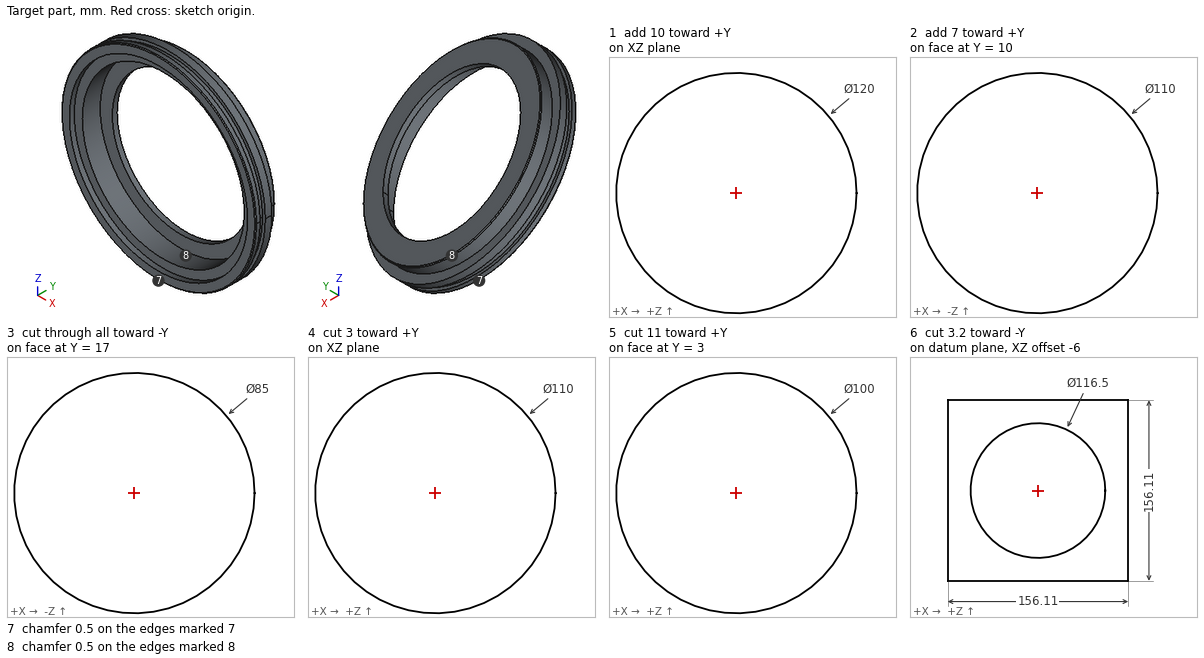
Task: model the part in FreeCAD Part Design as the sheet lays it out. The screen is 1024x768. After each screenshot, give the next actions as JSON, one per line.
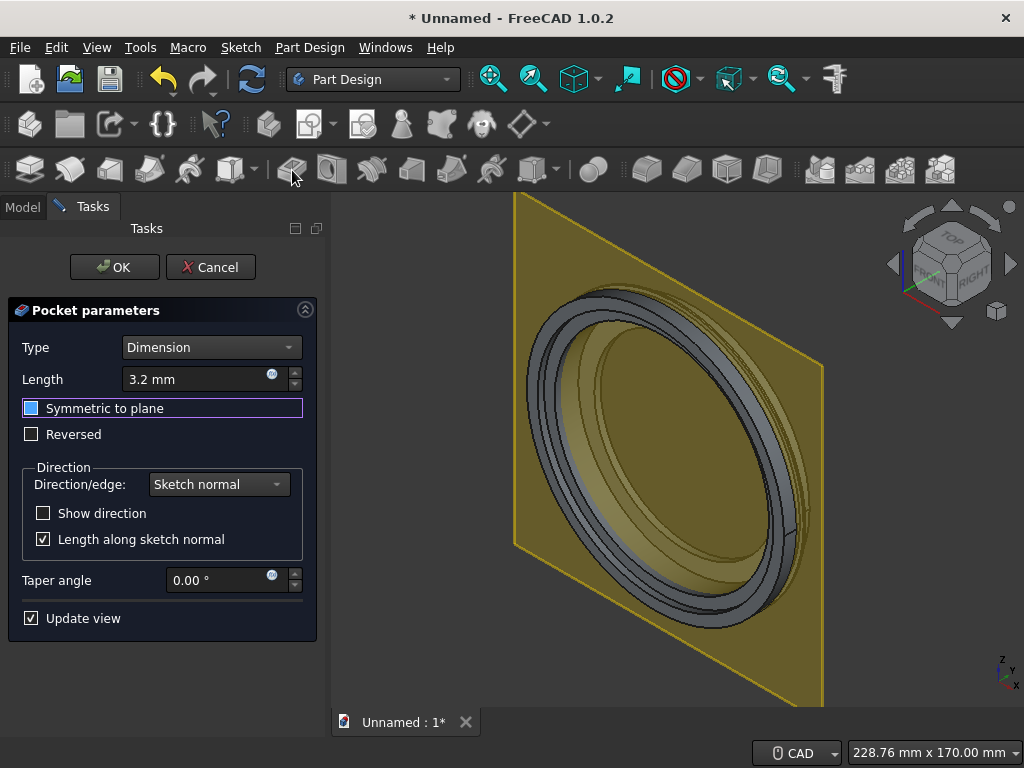
{"action": "left_click", "coordinate": [30, 434]}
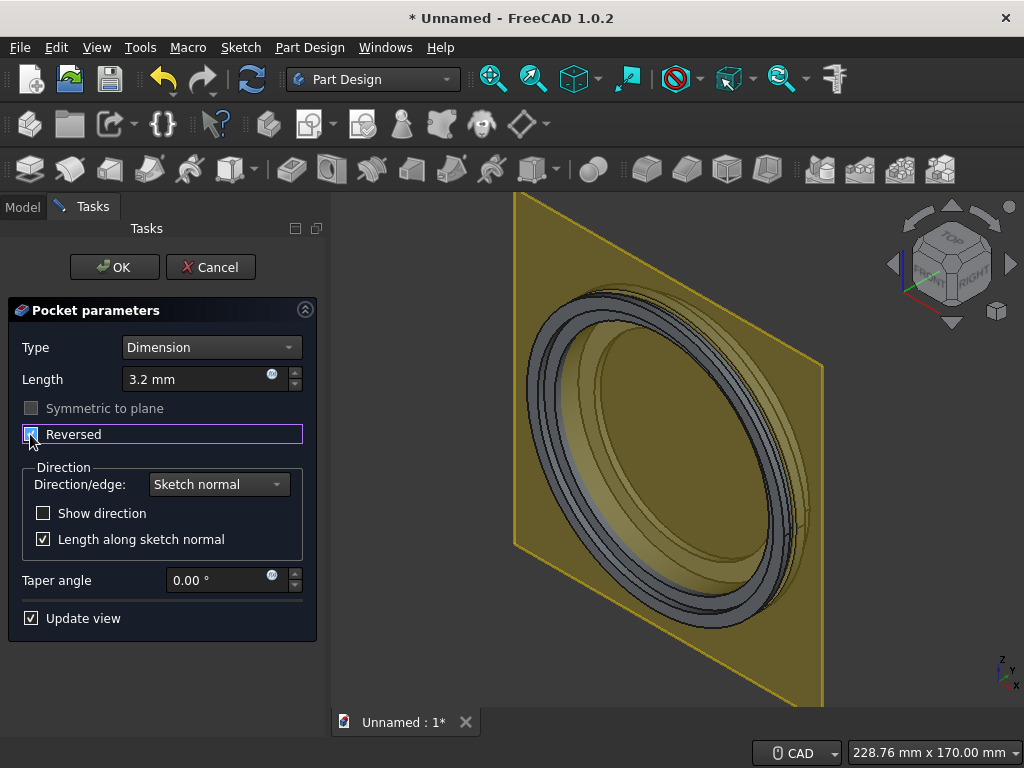
{"action": "left_click", "coordinate": [115, 267]}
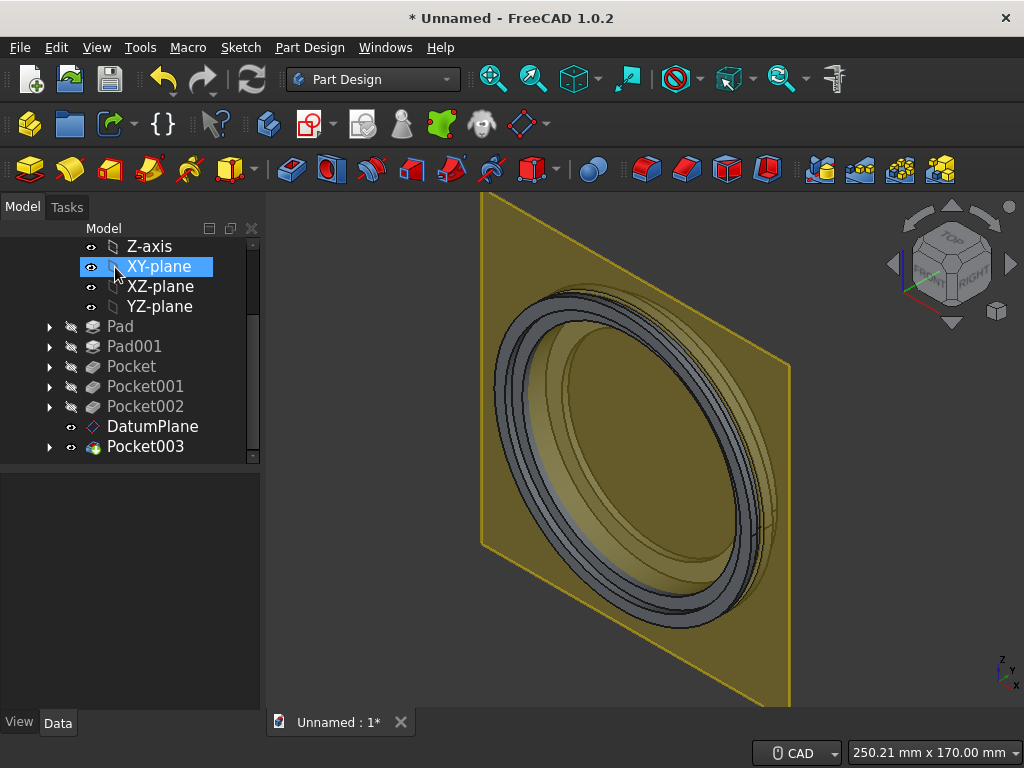
{"action": "left_click", "coordinate": [116, 427]}
{"action": "key", "text": "space"}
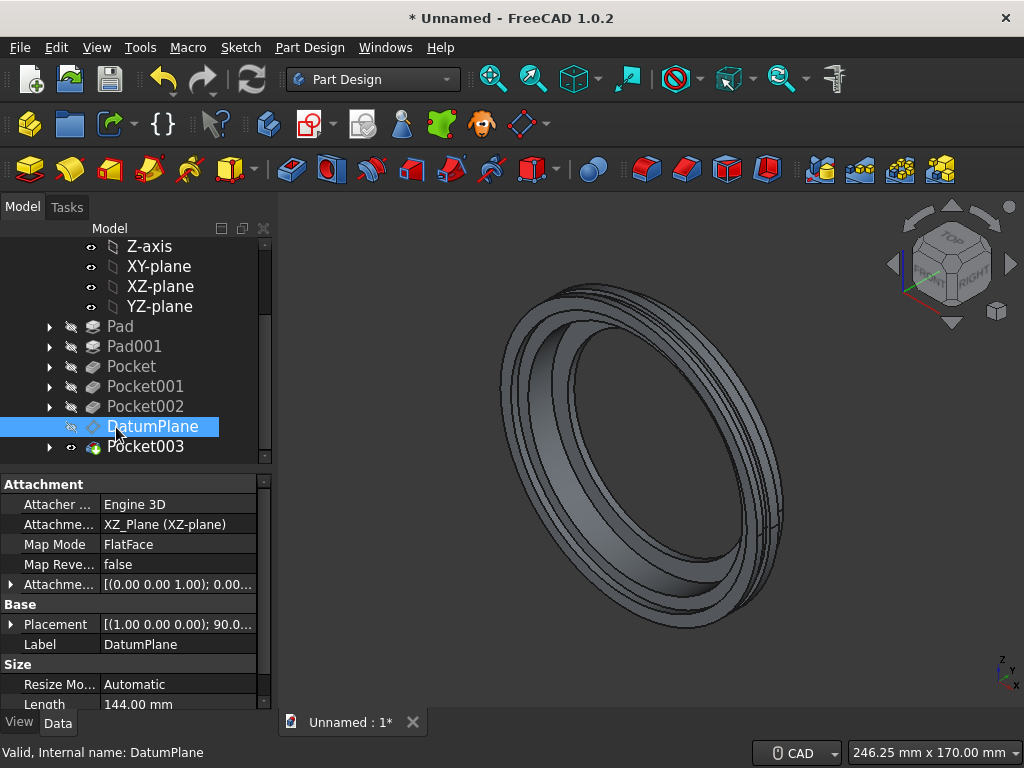
{"action": "left_click", "coordinate": [589, 297]}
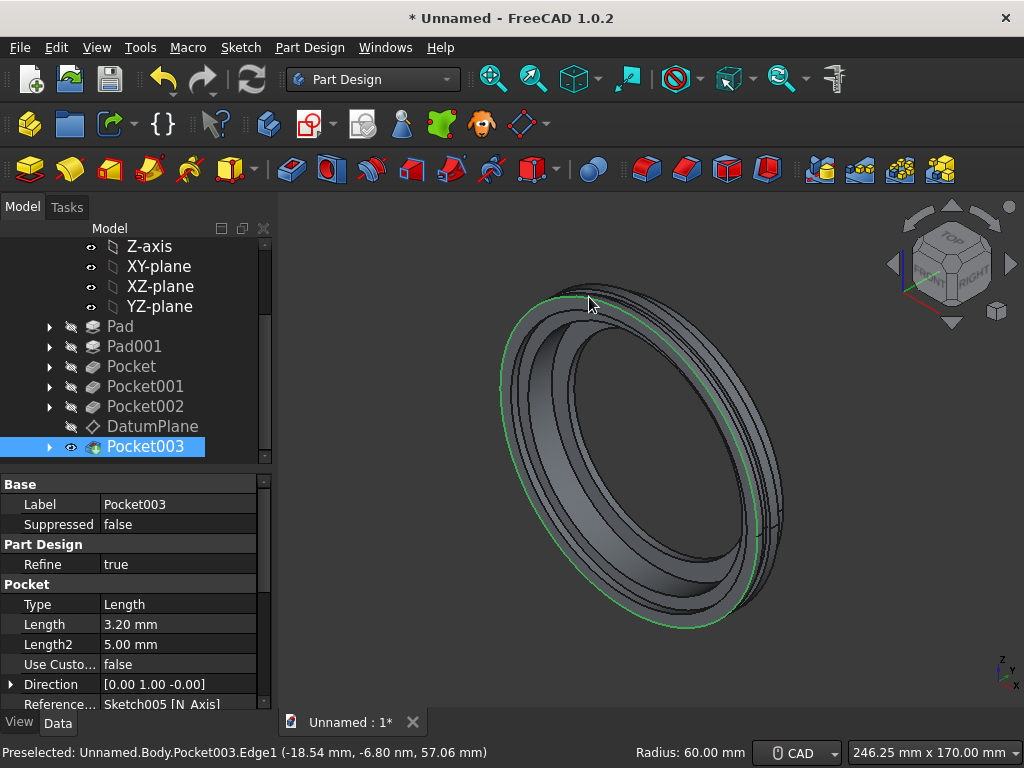
{"action": "left_click", "coordinate": [688, 170]}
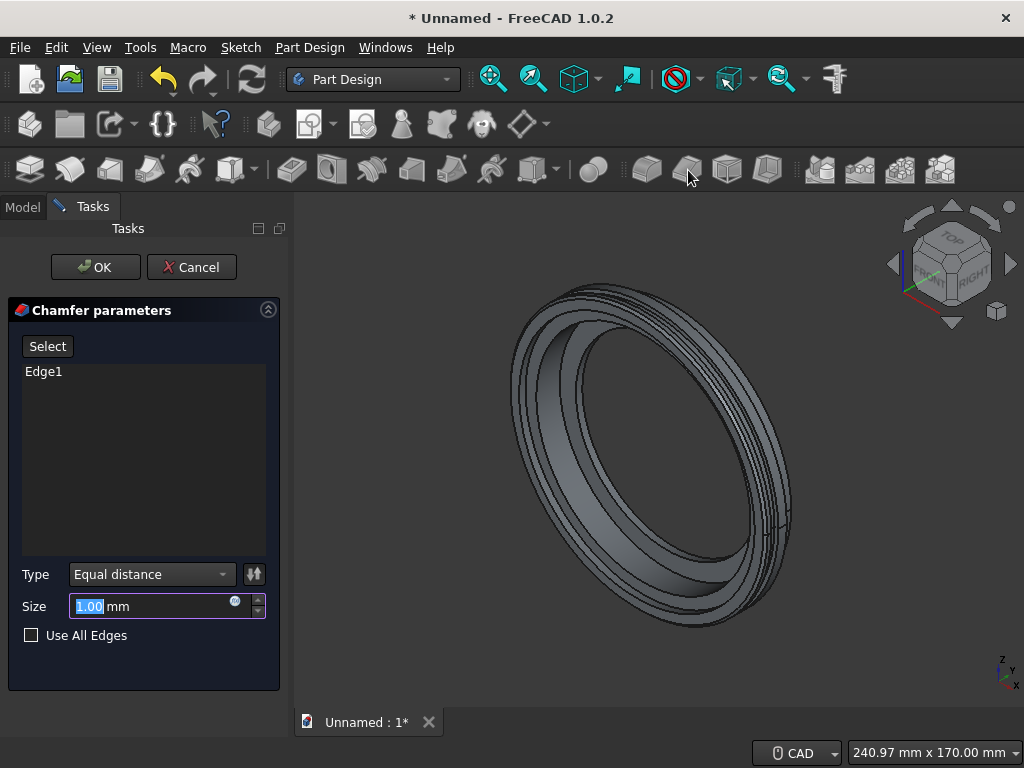
{"action": "type", "text": "0.5"}
{"action": "key", "text": "Tab"}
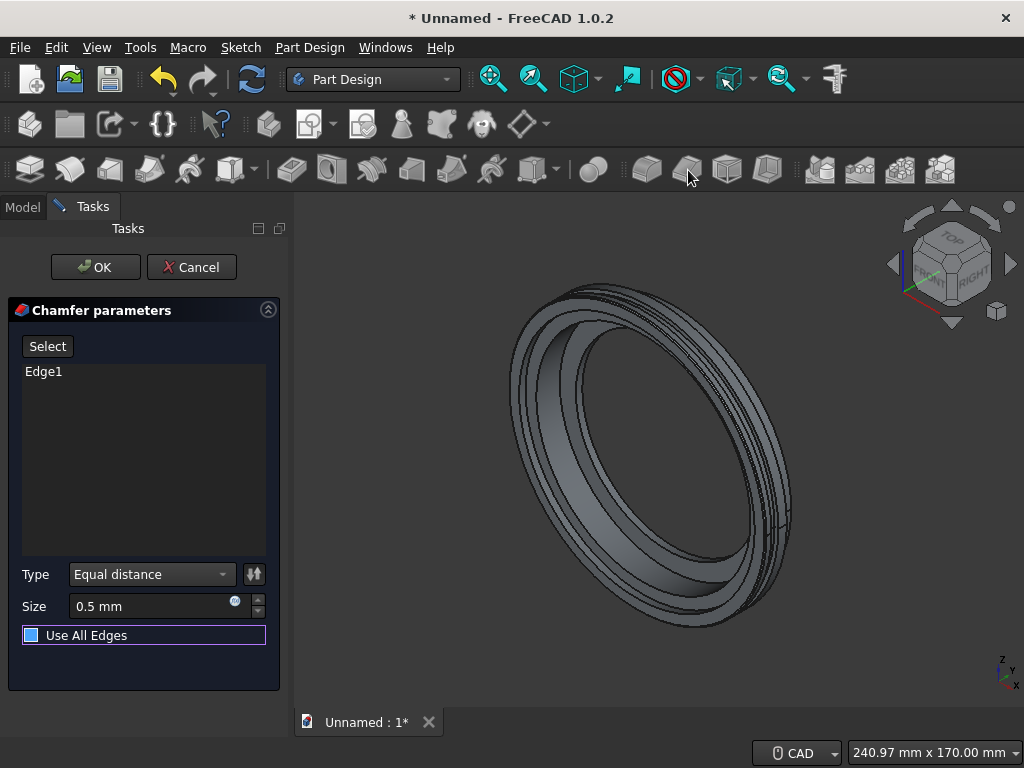
{"action": "left_click", "coordinate": [96, 267]}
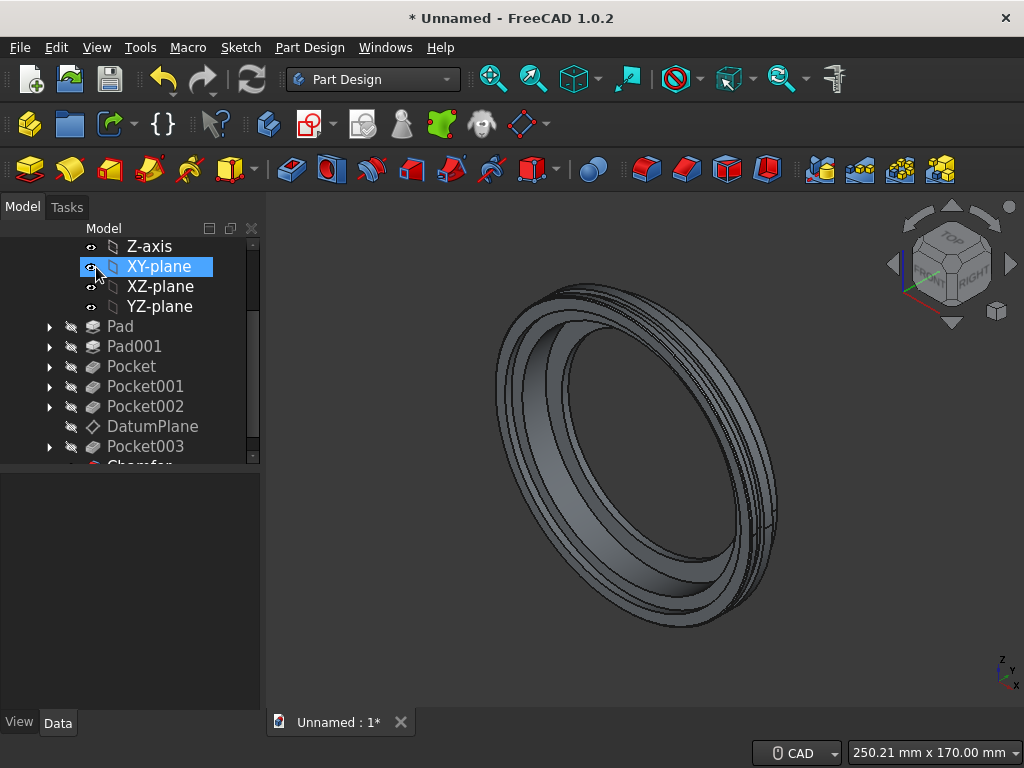
{"action": "key", "text": "2"}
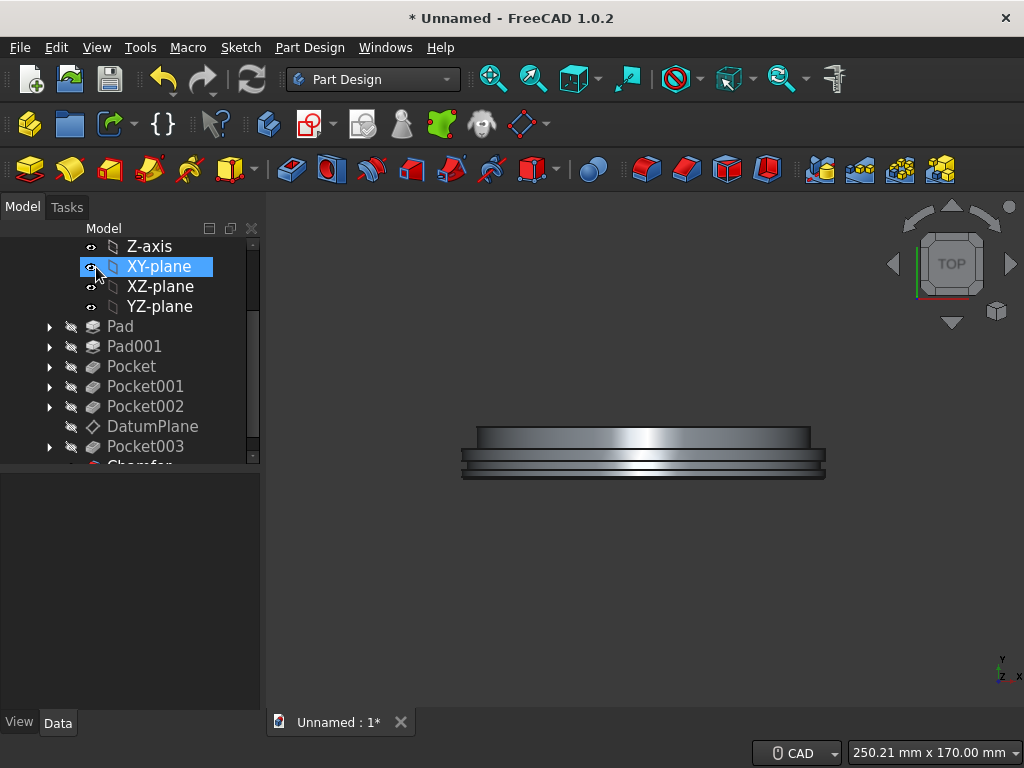
{"action": "left_click", "coordinate": [508, 426]}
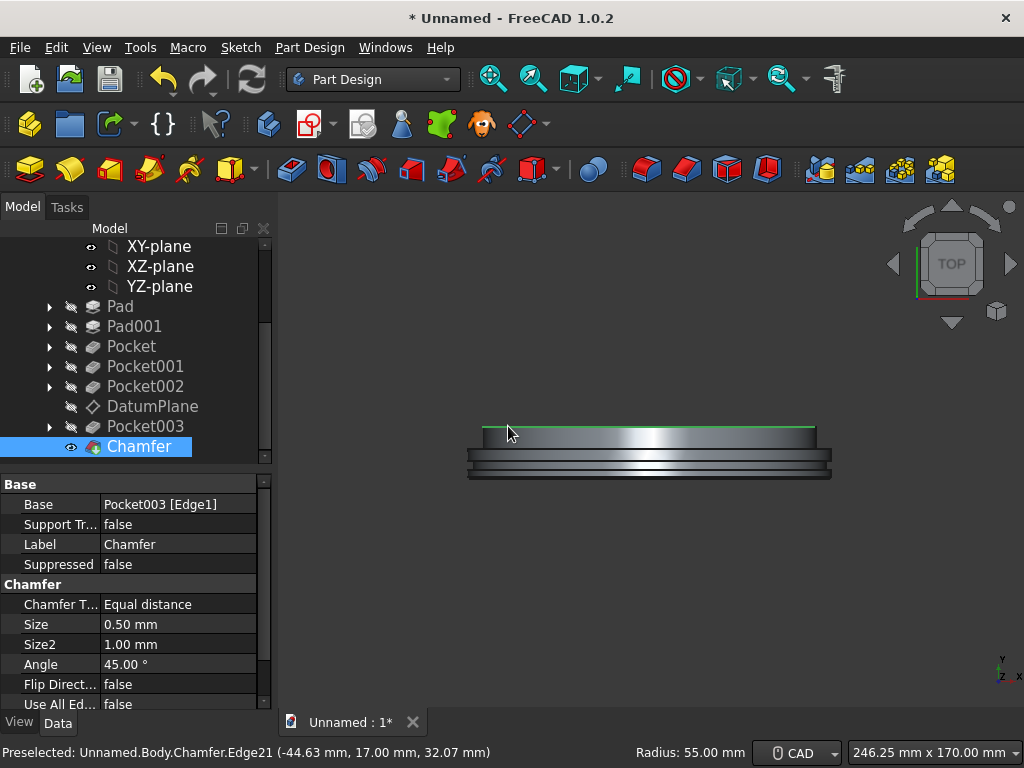
{"action": "left_click", "coordinate": [688, 170]}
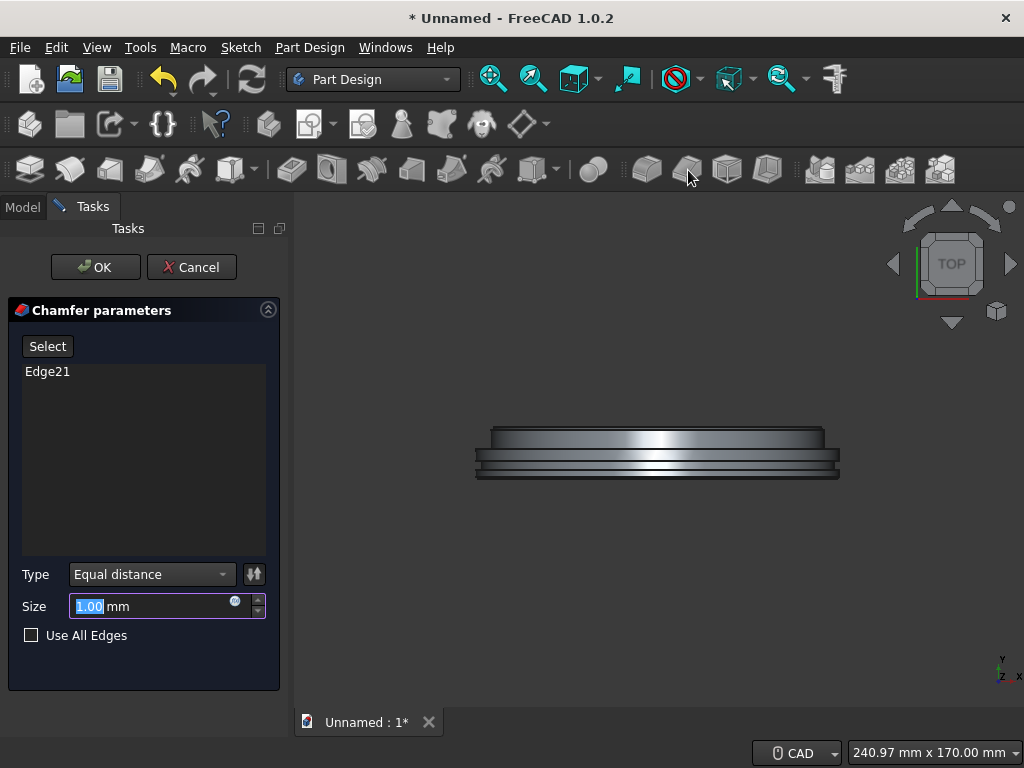
{"action": "type", "text": "0.5"}
{"action": "key", "text": "Tab"}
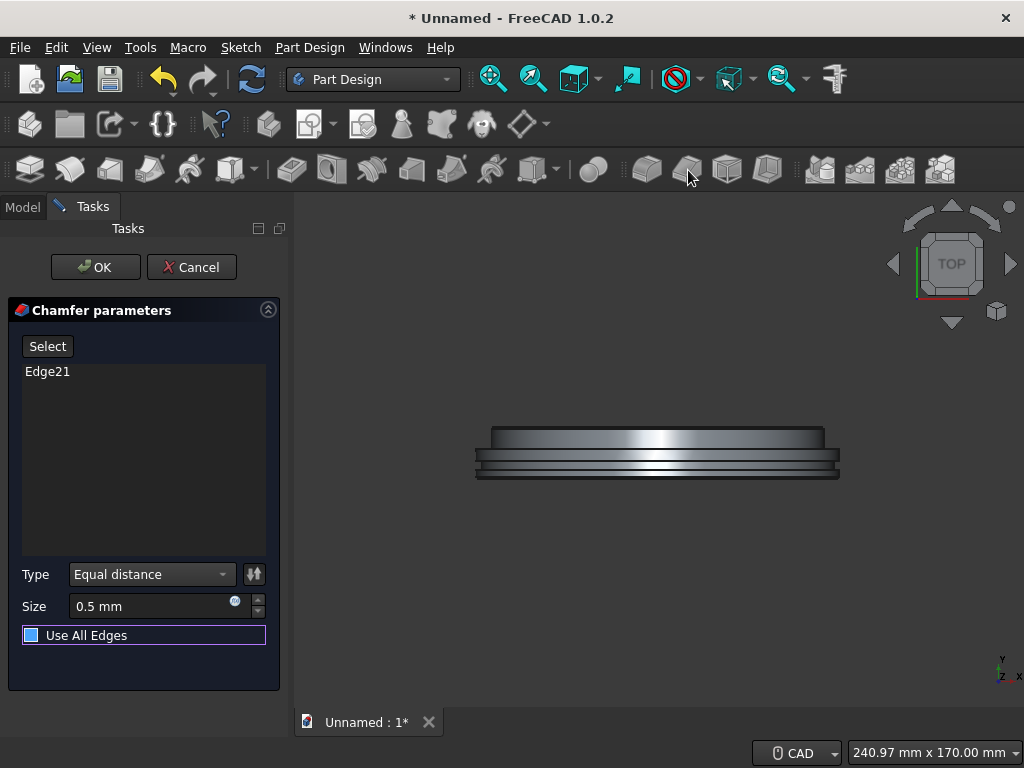
{"action": "left_click", "coordinate": [96, 267]}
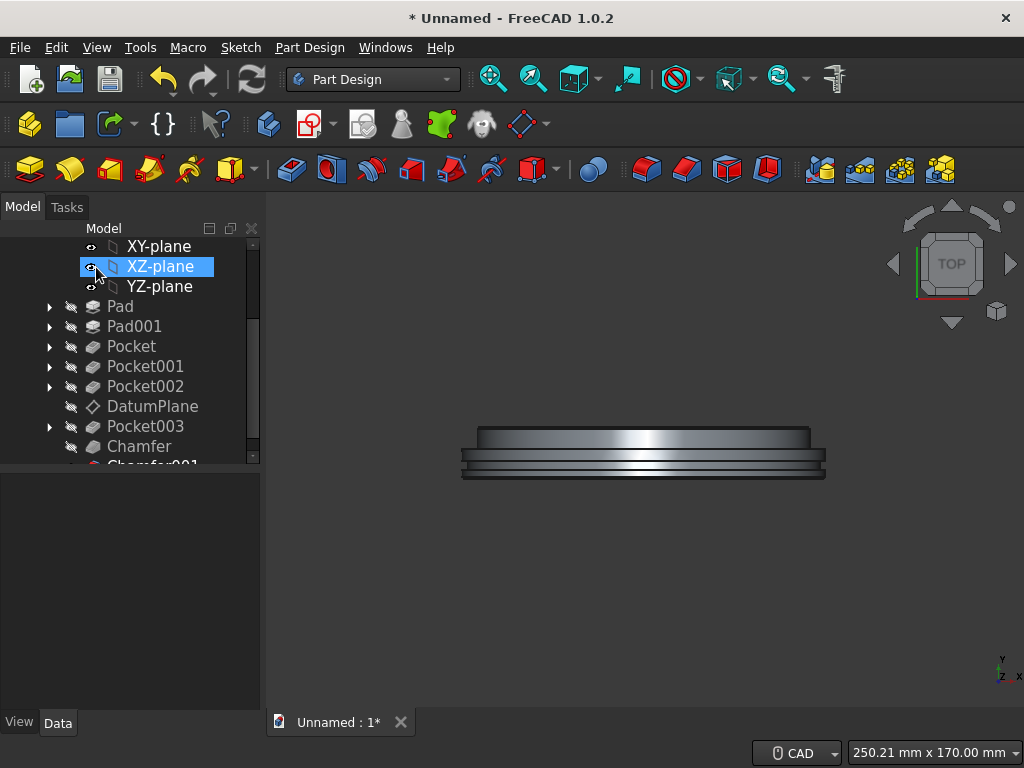
{"action": "key", "text": "0"}